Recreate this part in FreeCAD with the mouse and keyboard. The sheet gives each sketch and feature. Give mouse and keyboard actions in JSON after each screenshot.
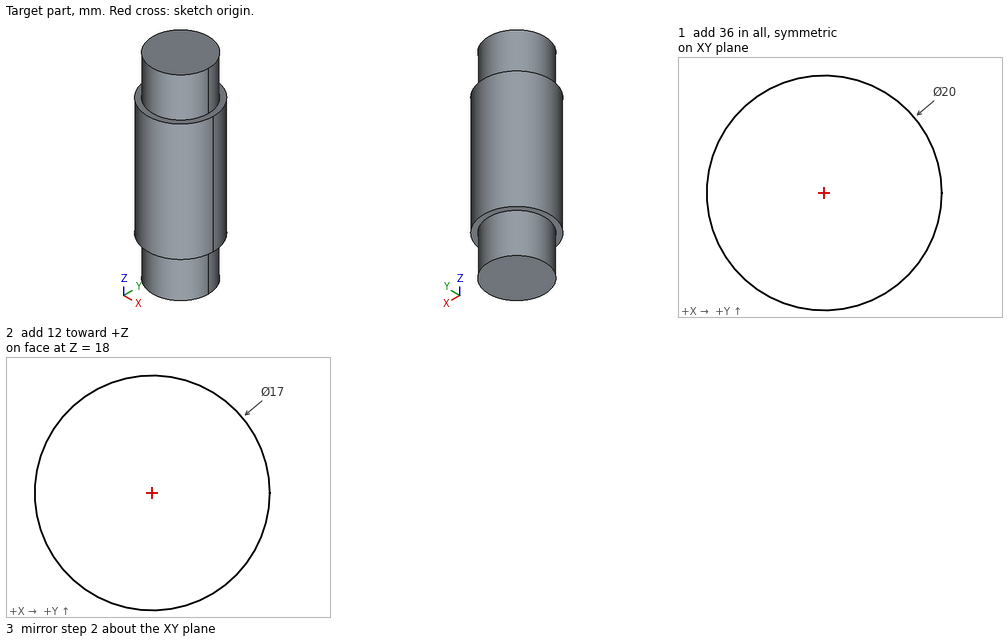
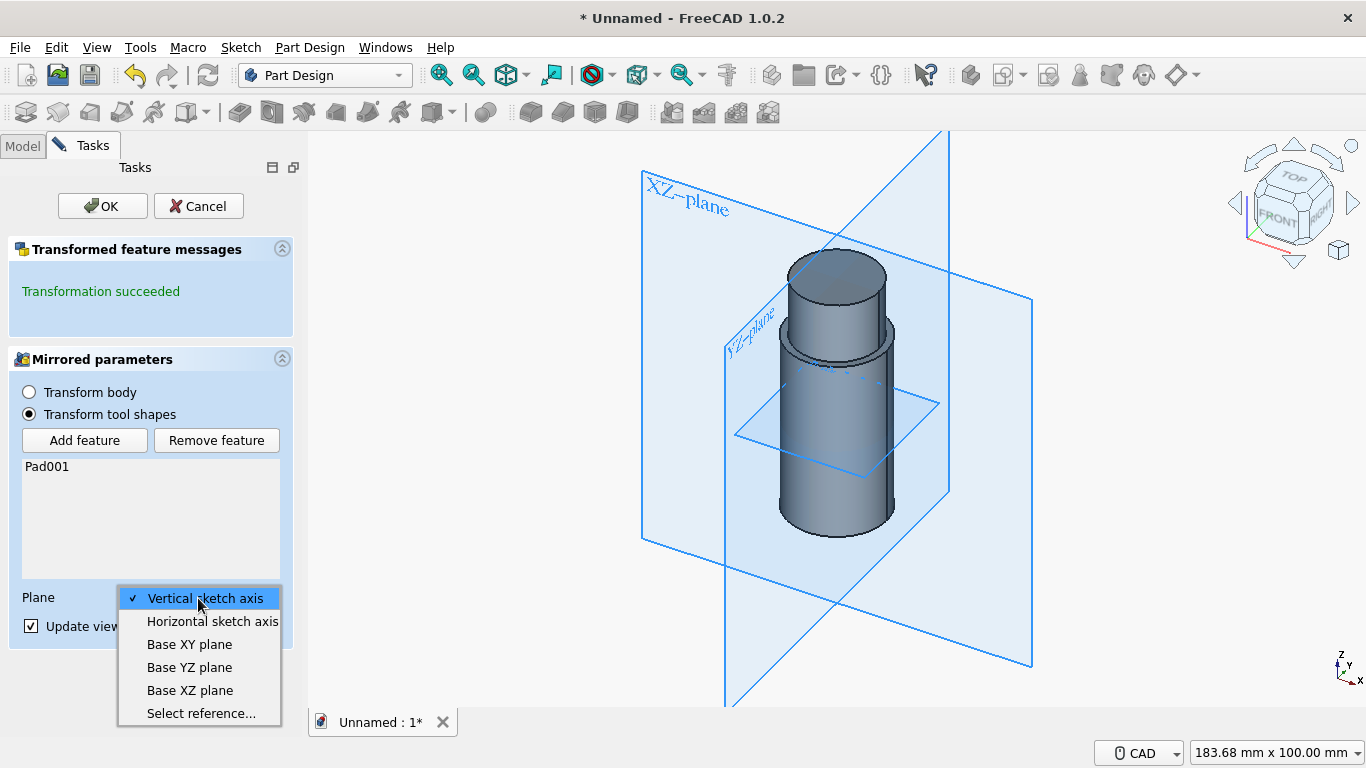
{"action": "left_click", "coordinate": [198, 644]}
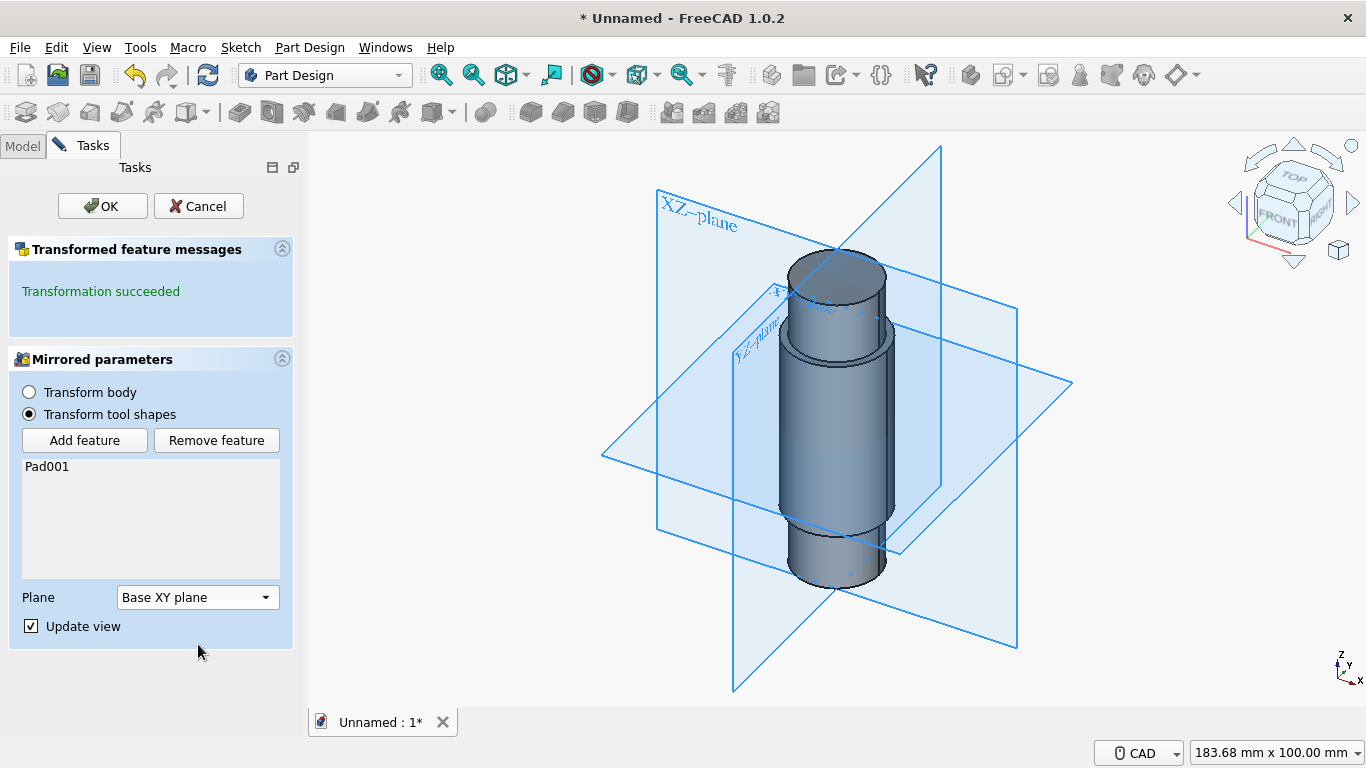
{"action": "left_click", "coordinate": [103, 206]}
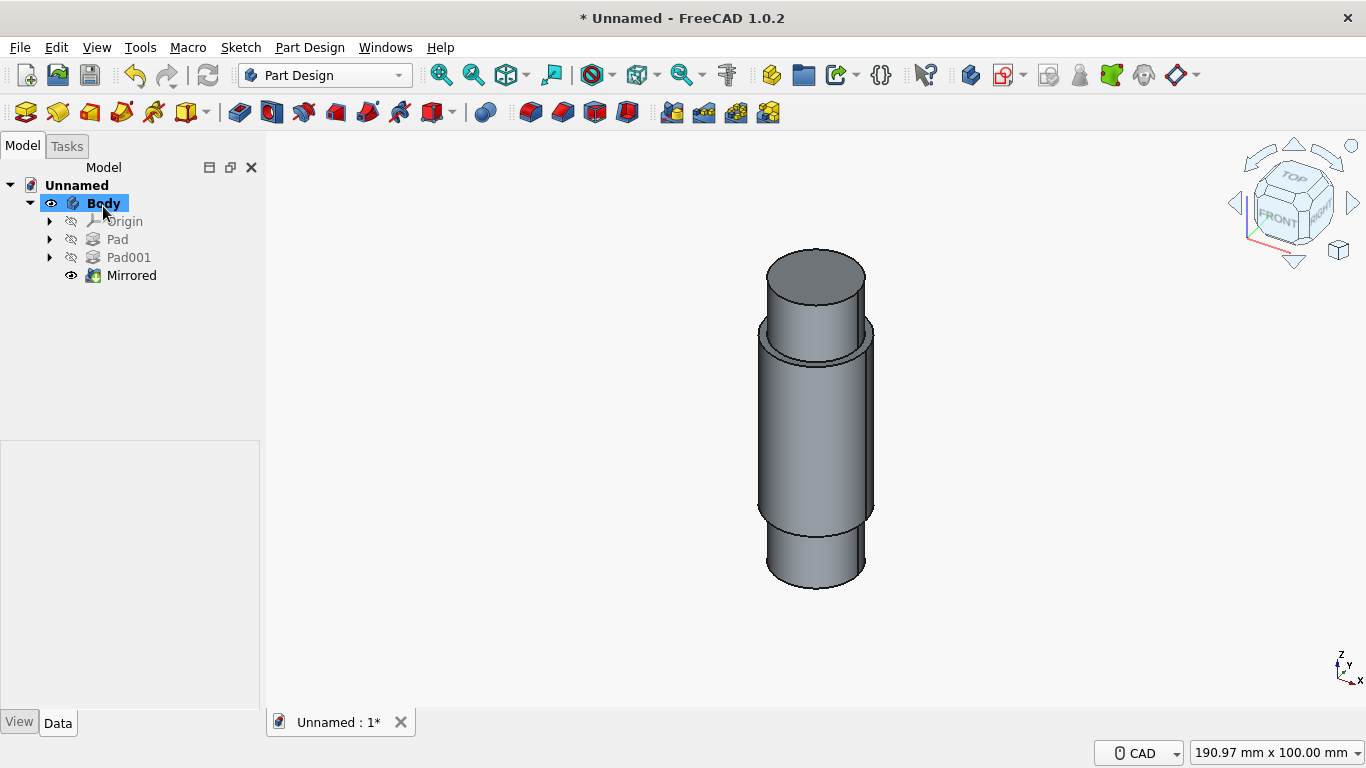
{"action": "key", "text": "0"}